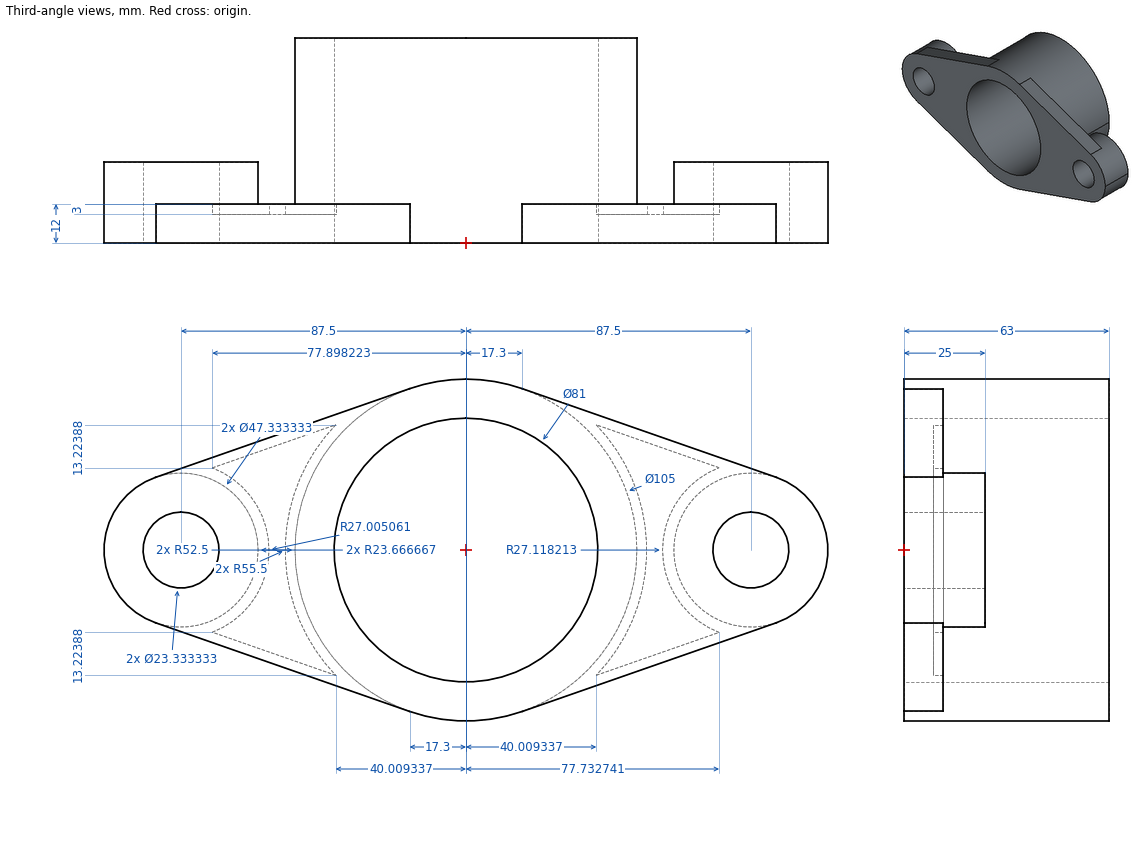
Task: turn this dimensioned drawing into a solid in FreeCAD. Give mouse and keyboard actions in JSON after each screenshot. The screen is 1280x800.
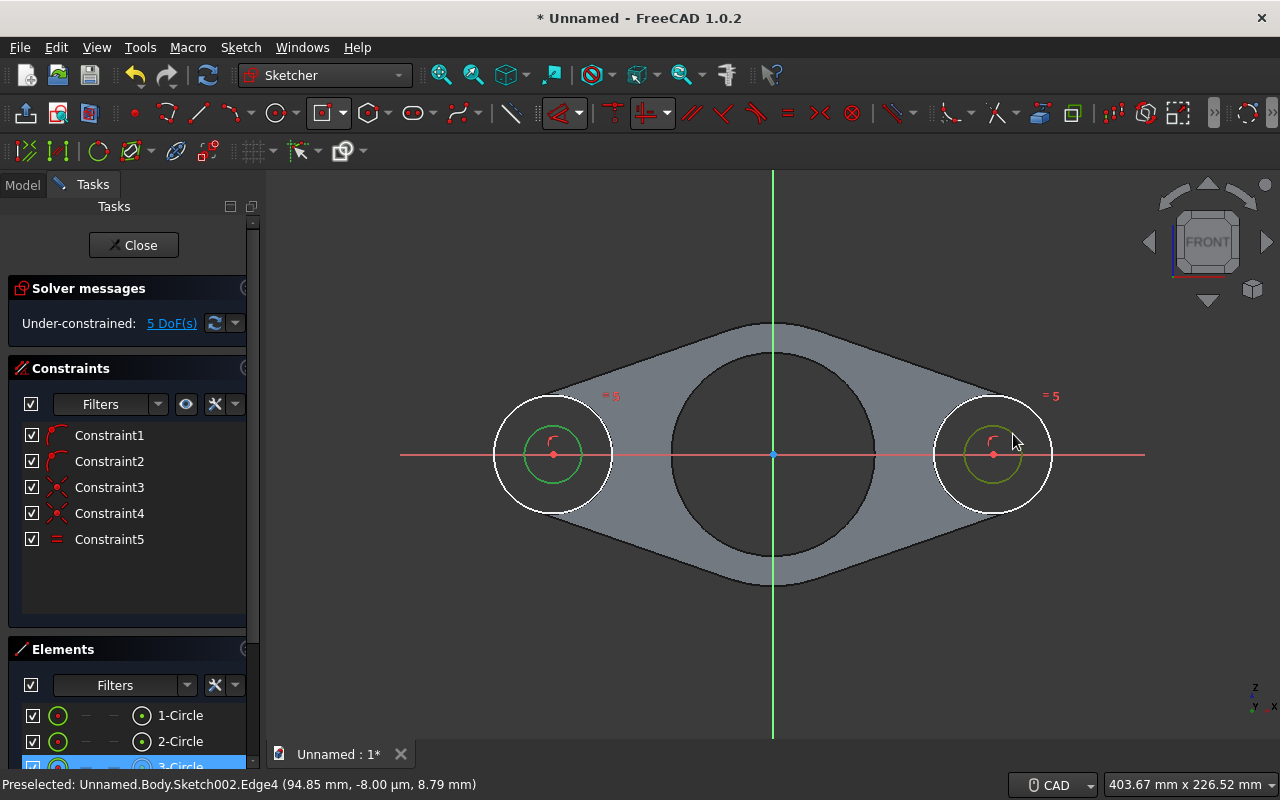
{"action": "key", "text": "e"}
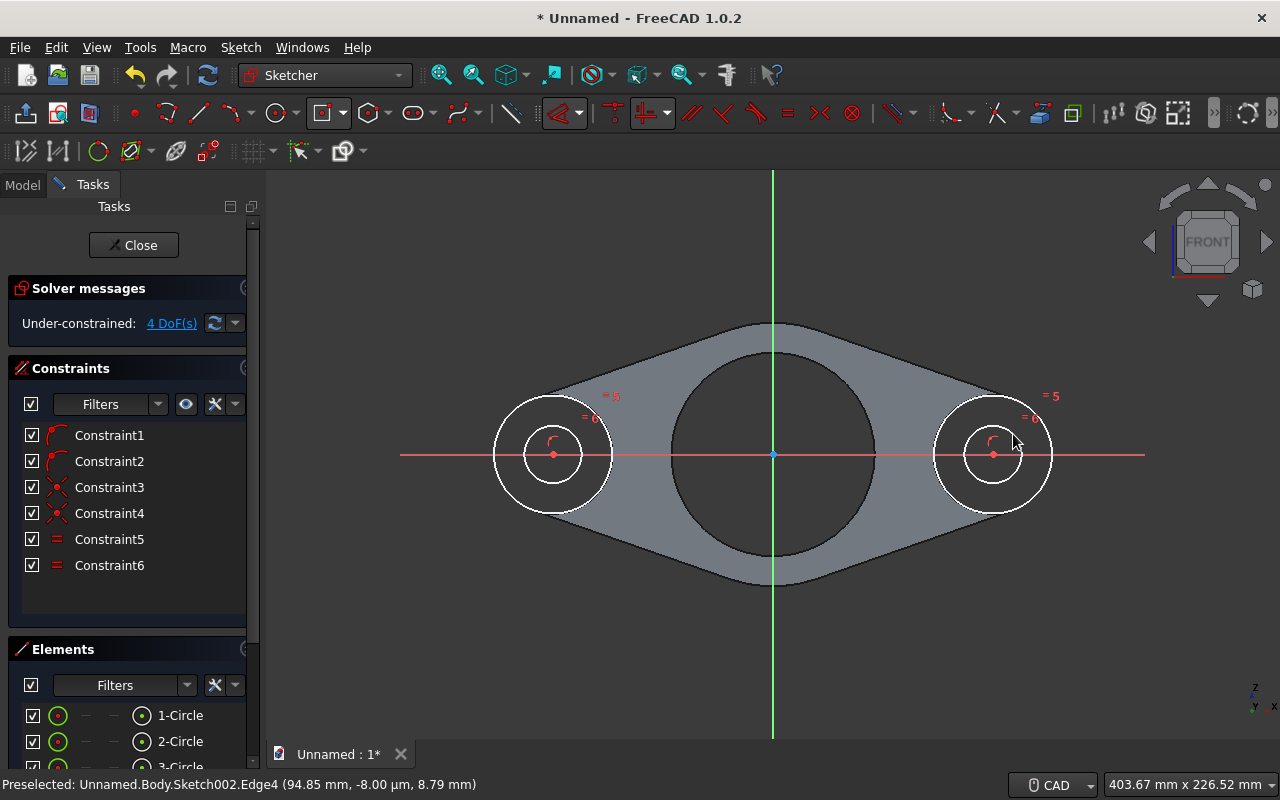
{"action": "left_click", "coordinate": [511, 413]}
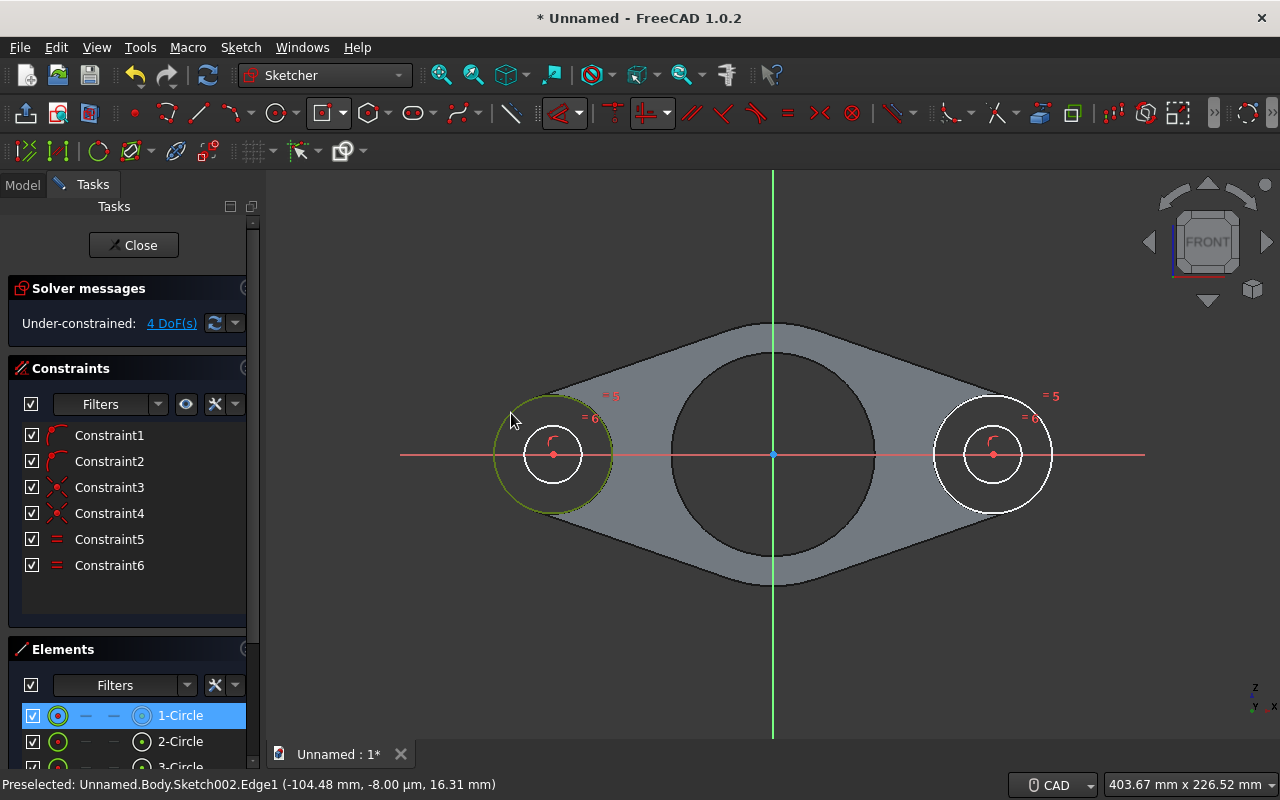
{"action": "key", "text": "k o"}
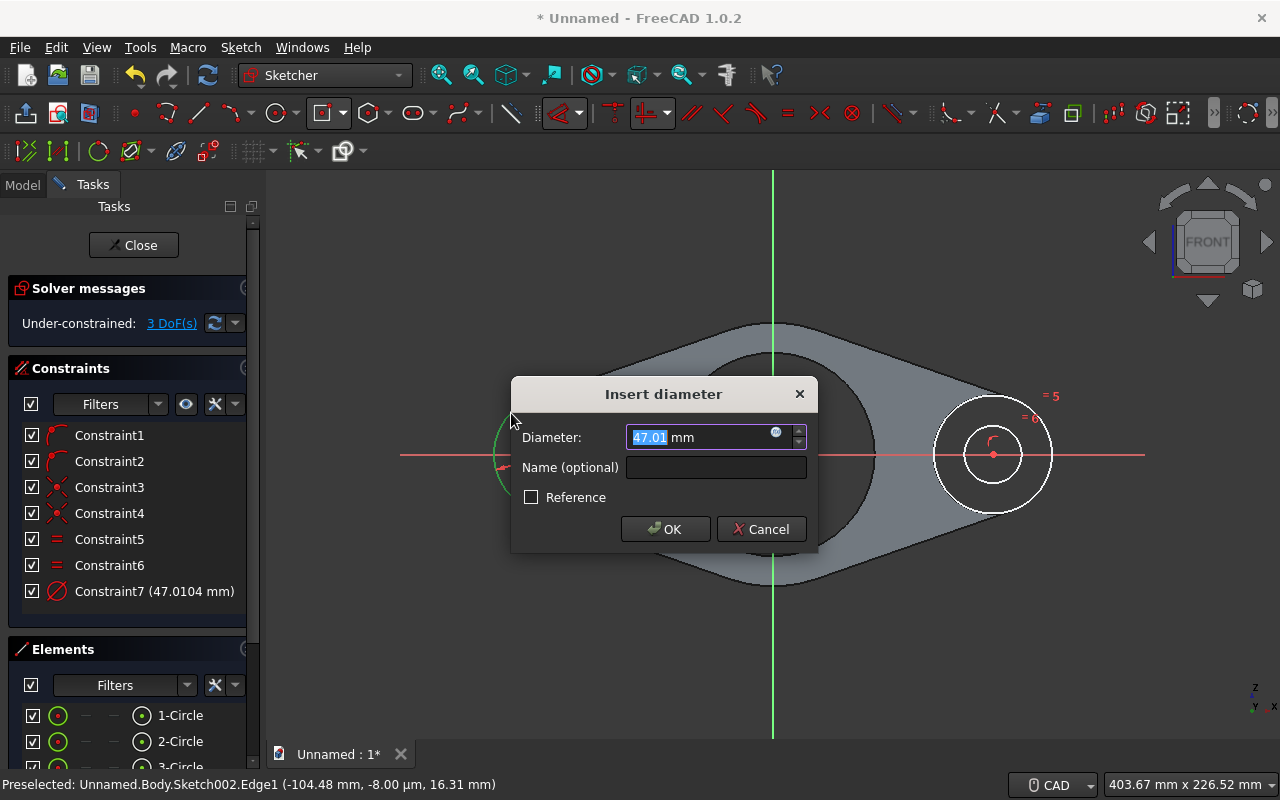
{"action": "type", "text": "47.333333"}
{"action": "key", "text": "Return"}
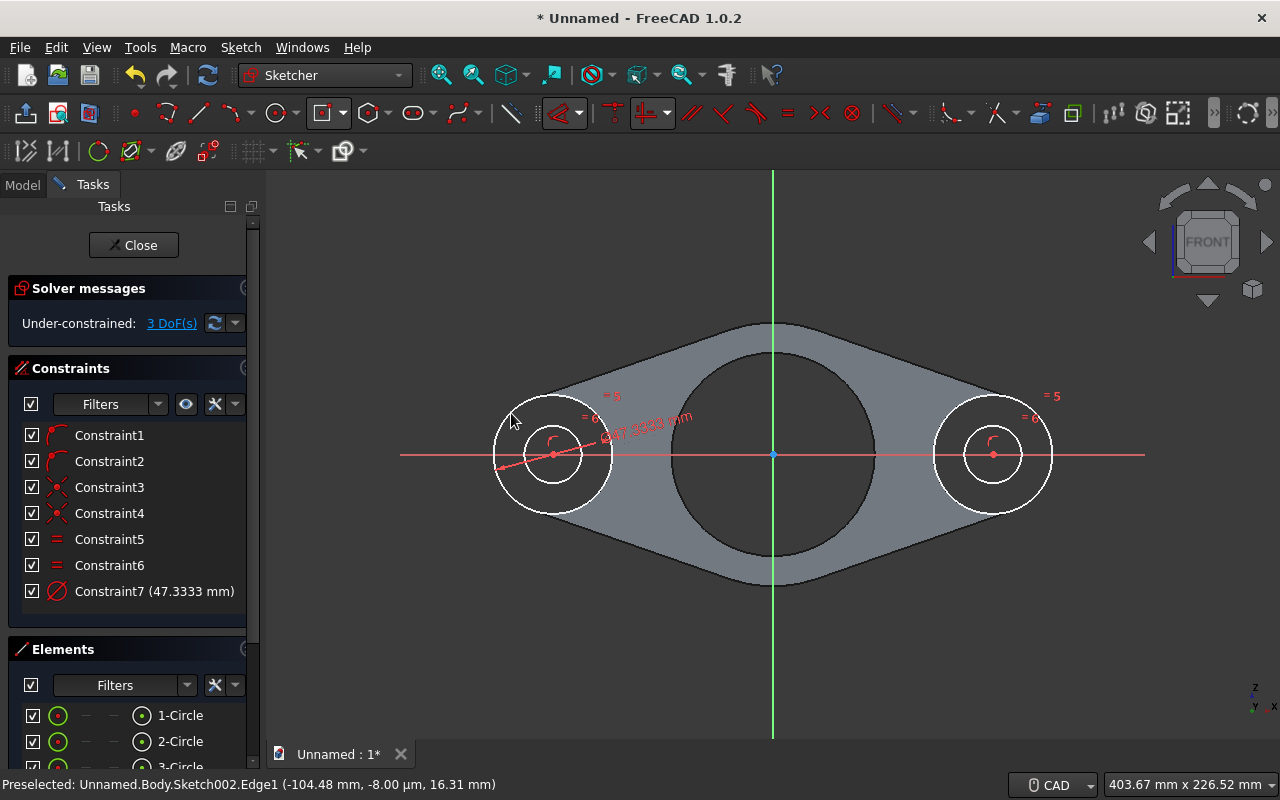
{"action": "left_click", "coordinate": [573, 434]}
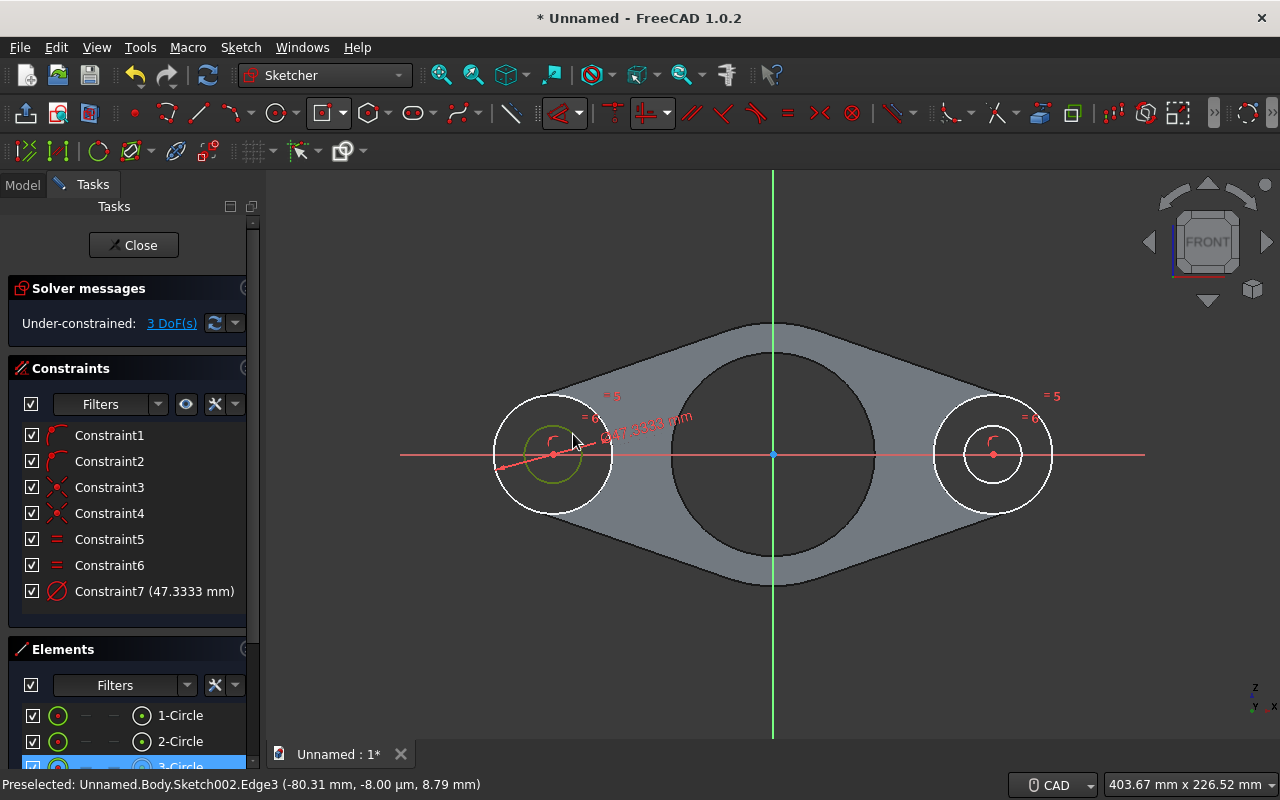
{"action": "key", "text": "k o"}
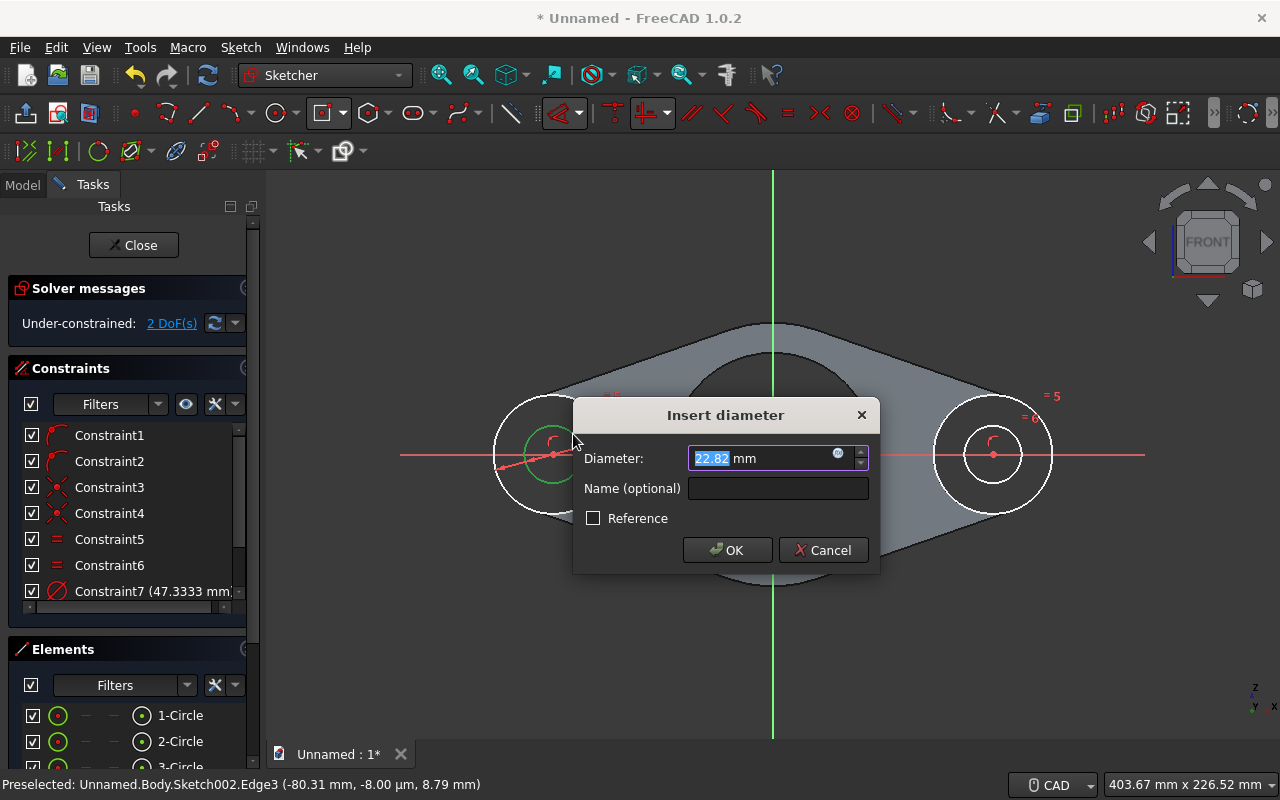
{"action": "type", "text": "23.333333"}
{"action": "key", "text": "Return"}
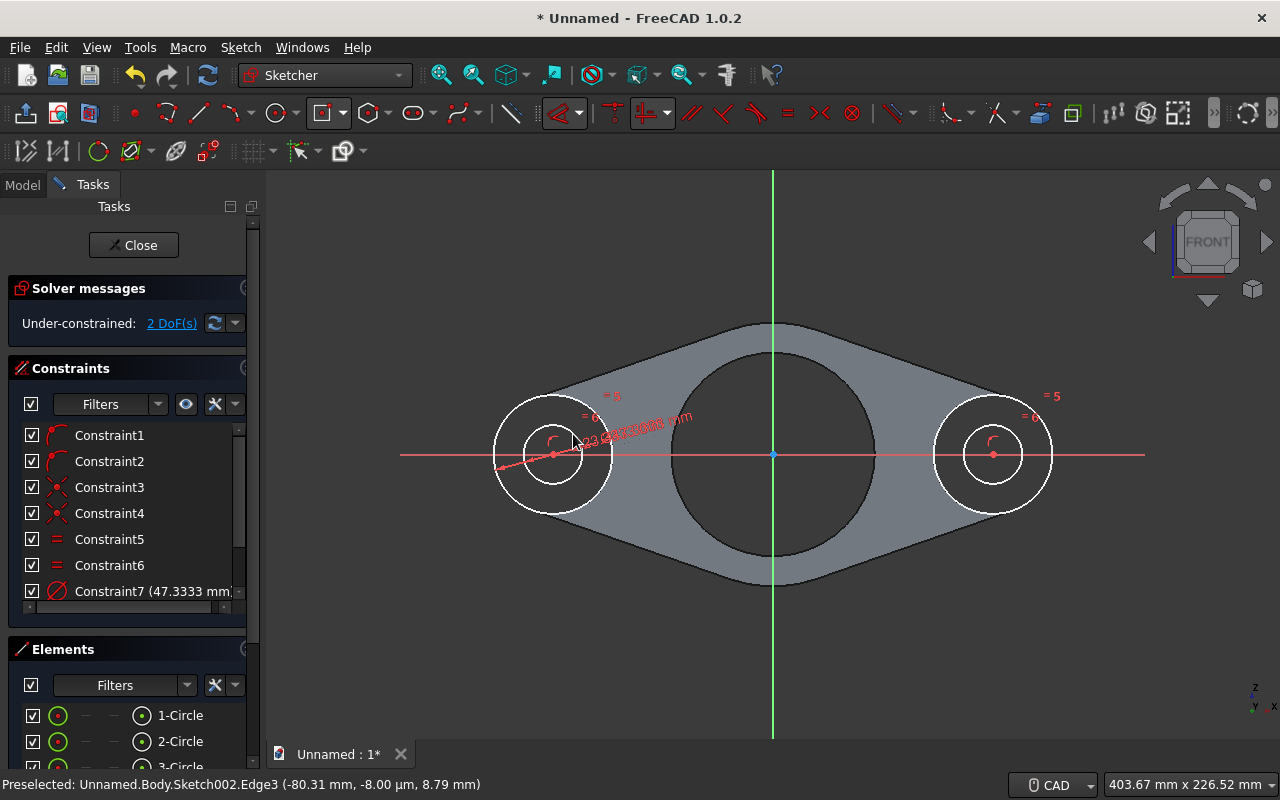
{"action": "left_click", "coordinate": [553, 455]}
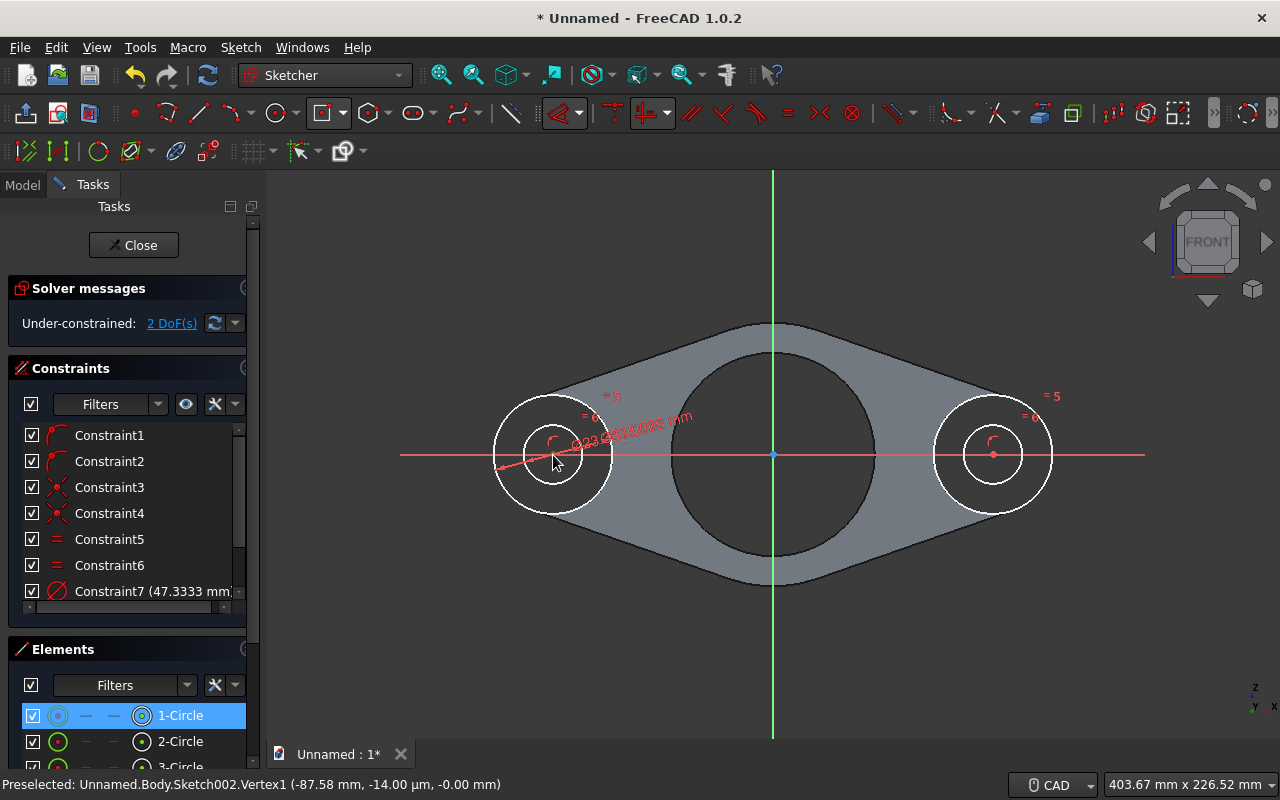
{"action": "key", "text": "l"}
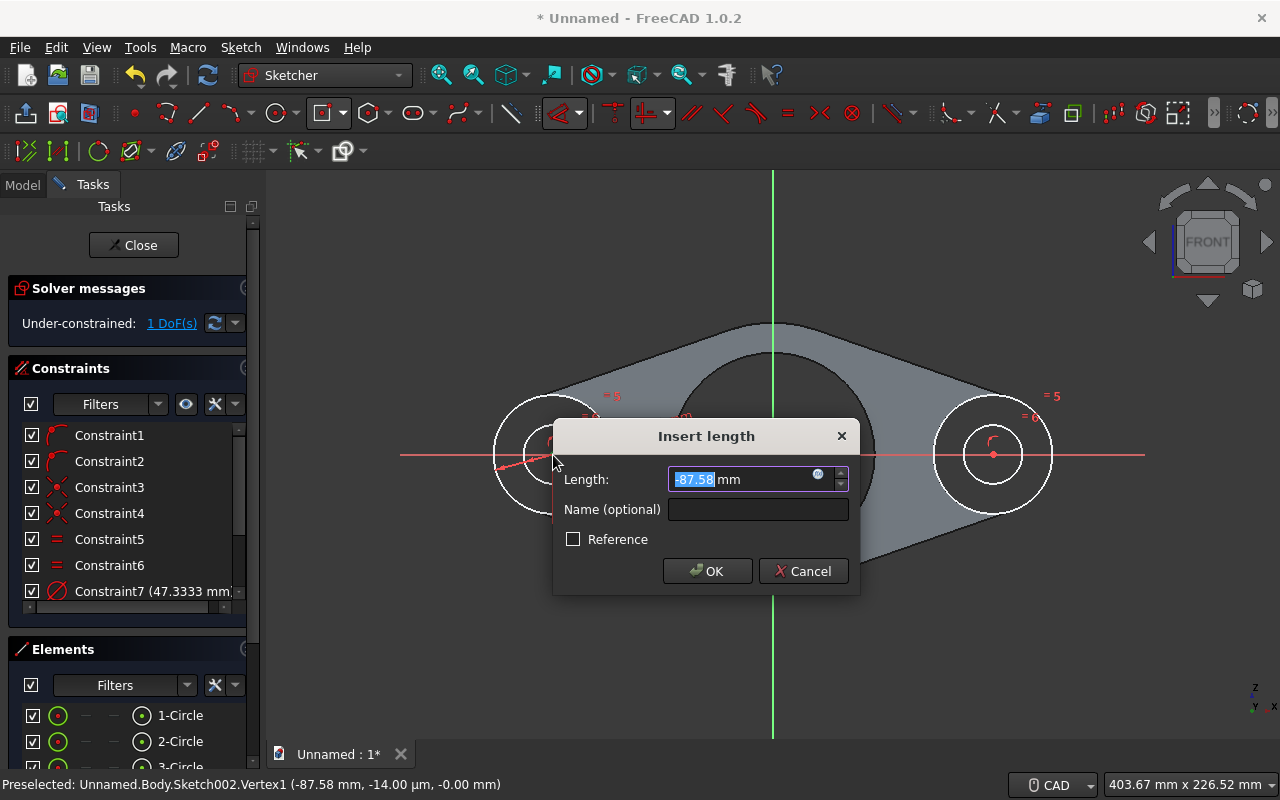
{"action": "type", "text": "-87.5"}
{"action": "key", "text": "Return"}